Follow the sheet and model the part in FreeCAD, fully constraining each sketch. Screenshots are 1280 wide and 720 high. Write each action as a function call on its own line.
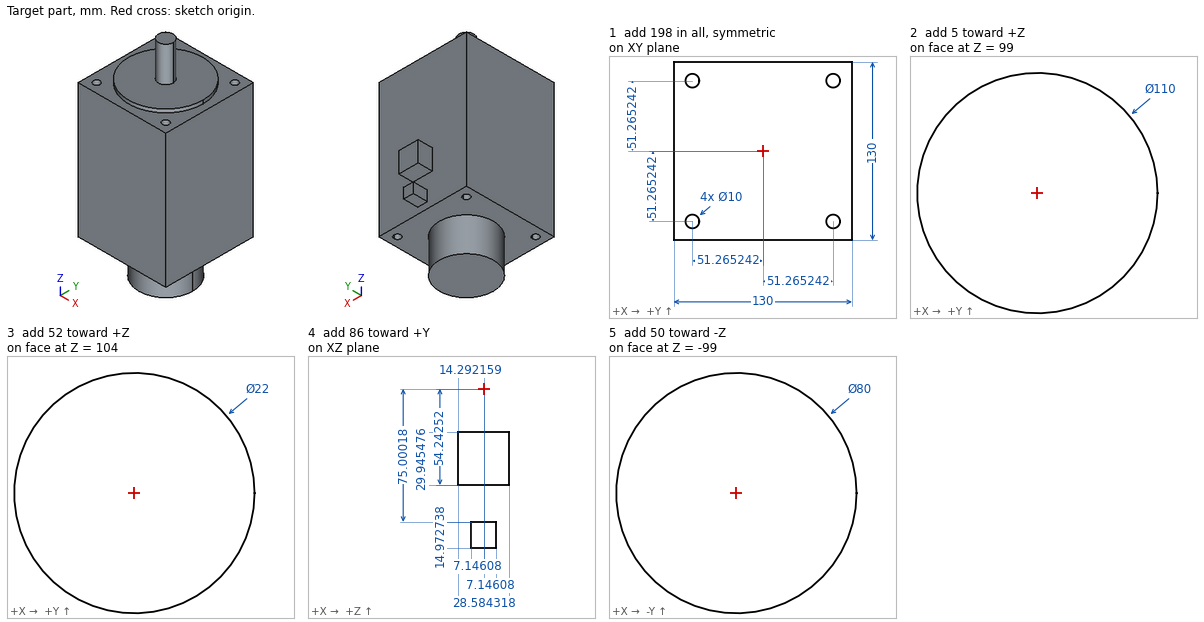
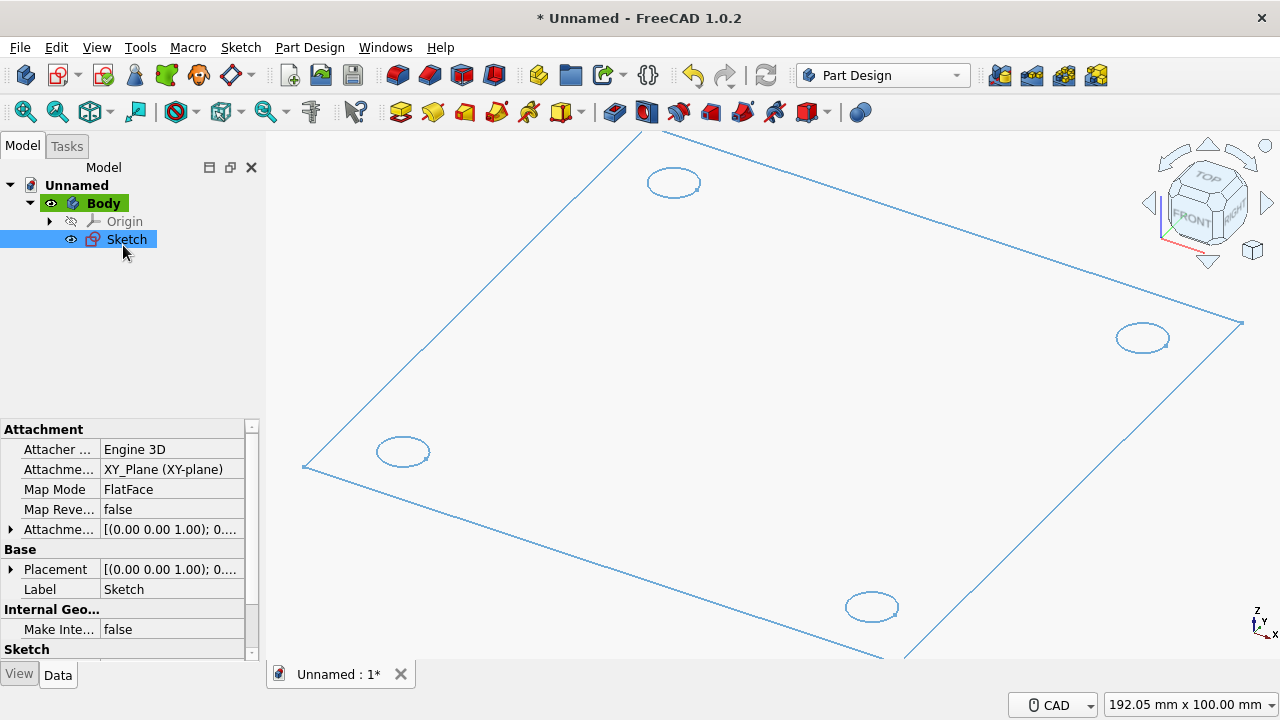
click(402, 112)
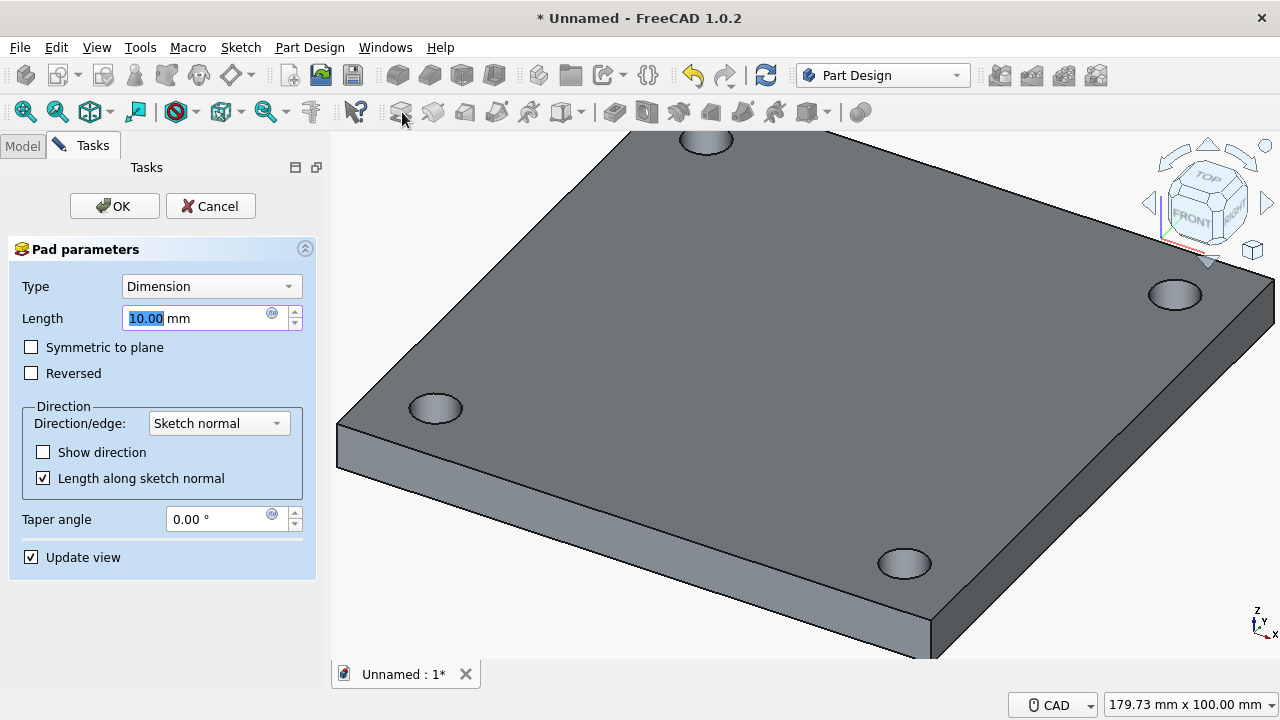
text(198)
key(Tab)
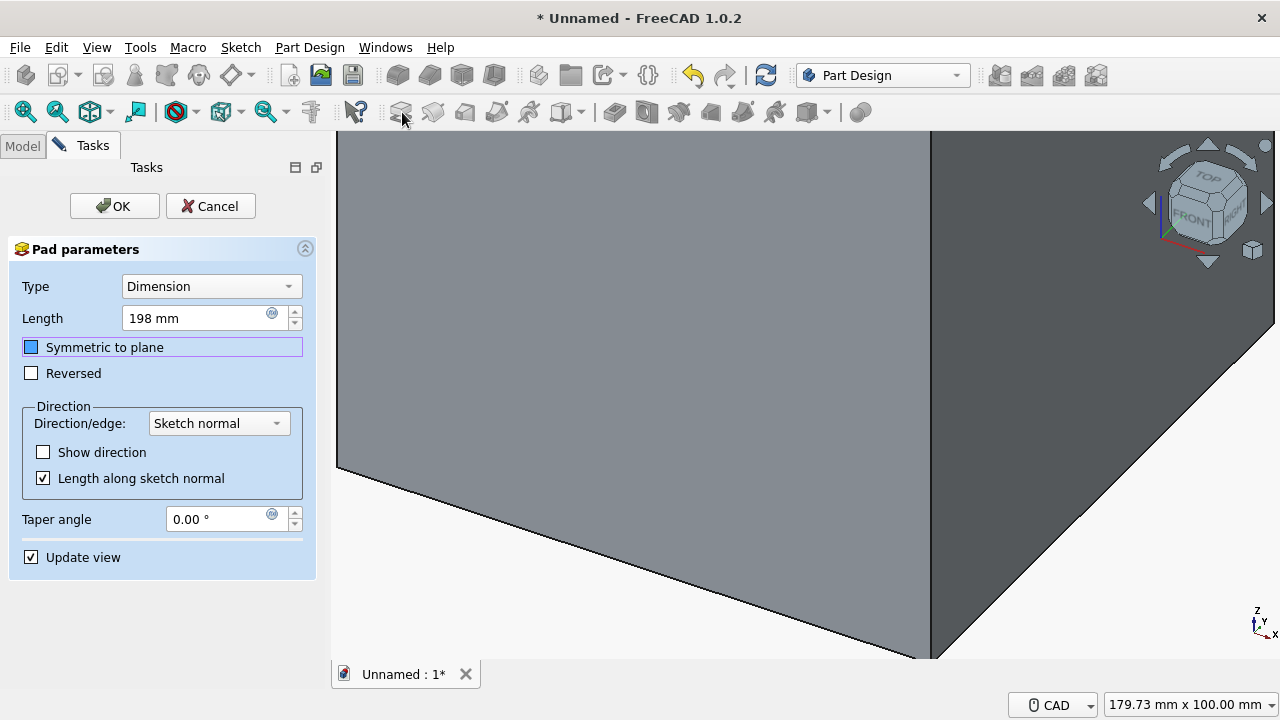
click(30, 347)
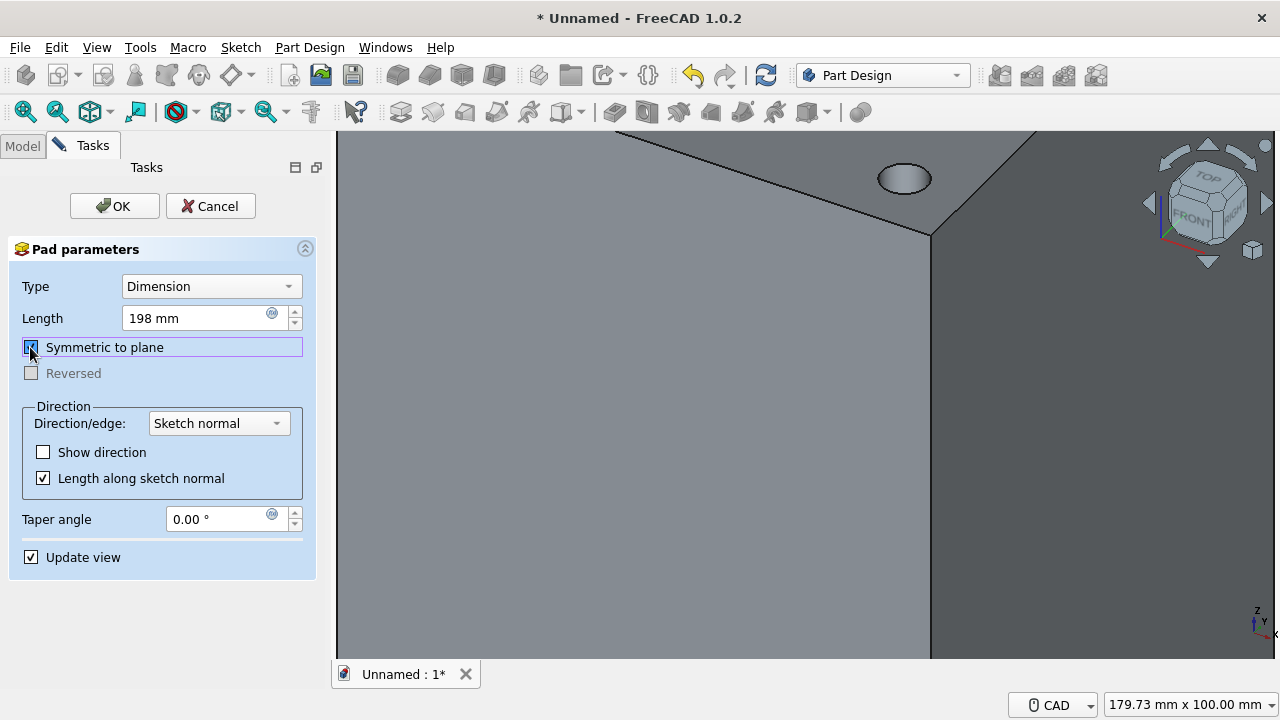
click(115, 206)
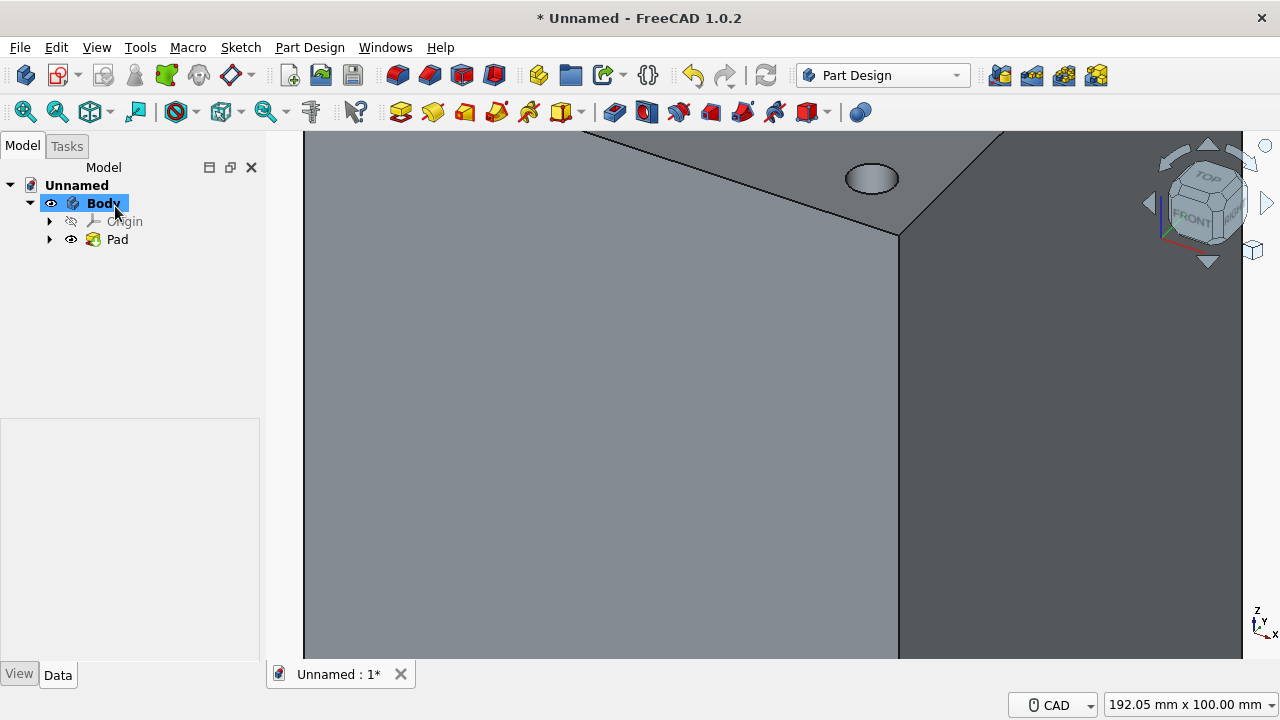
click(26, 112)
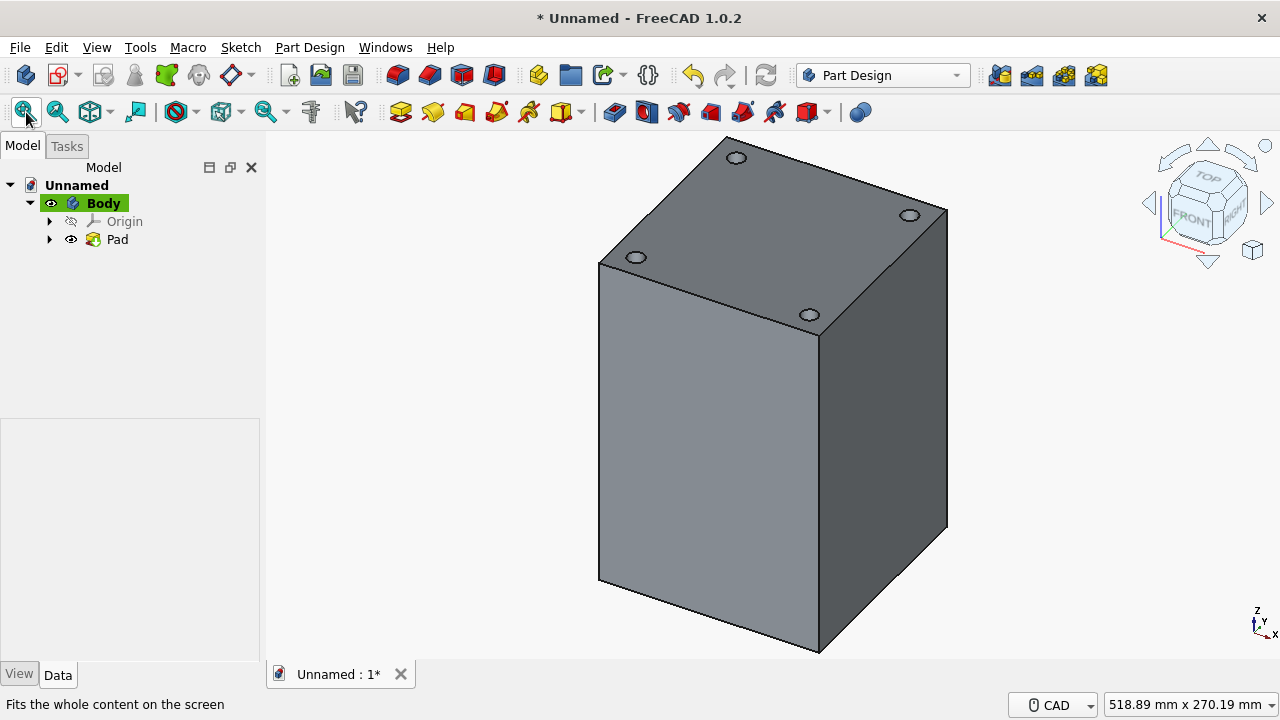
click(773, 236)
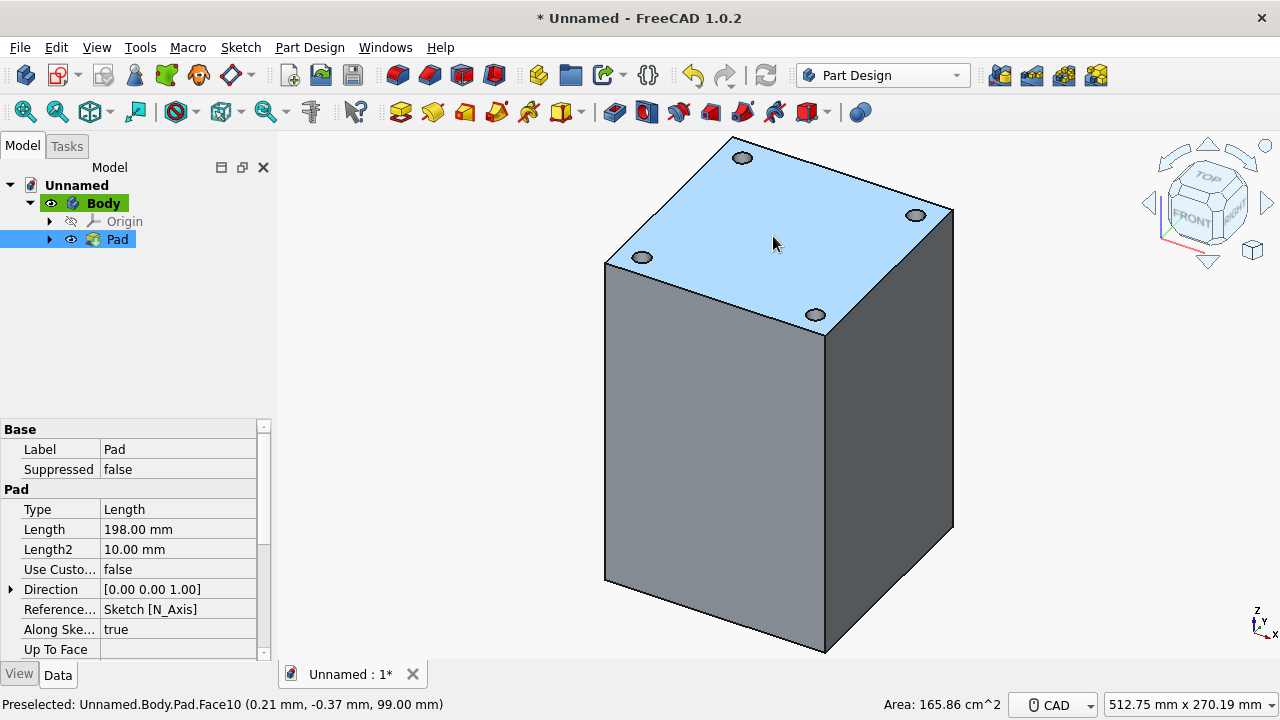
click(58, 76)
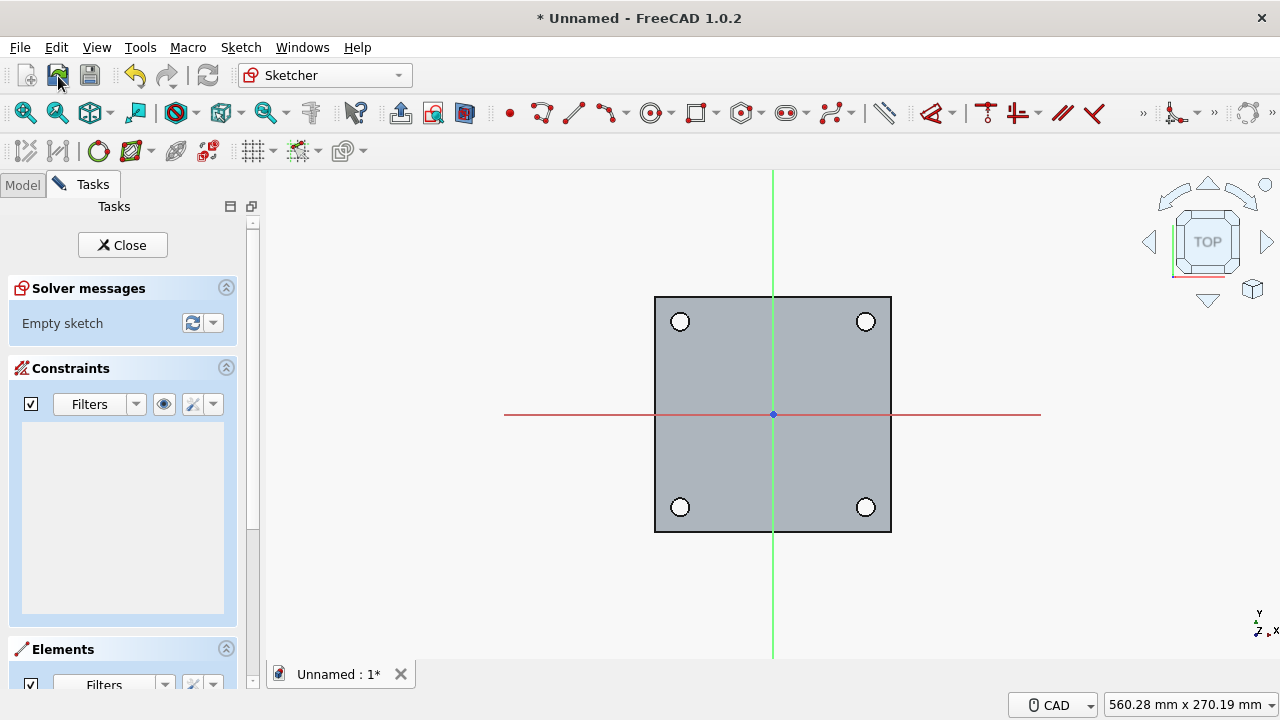
scroll(912, 414, up, 2)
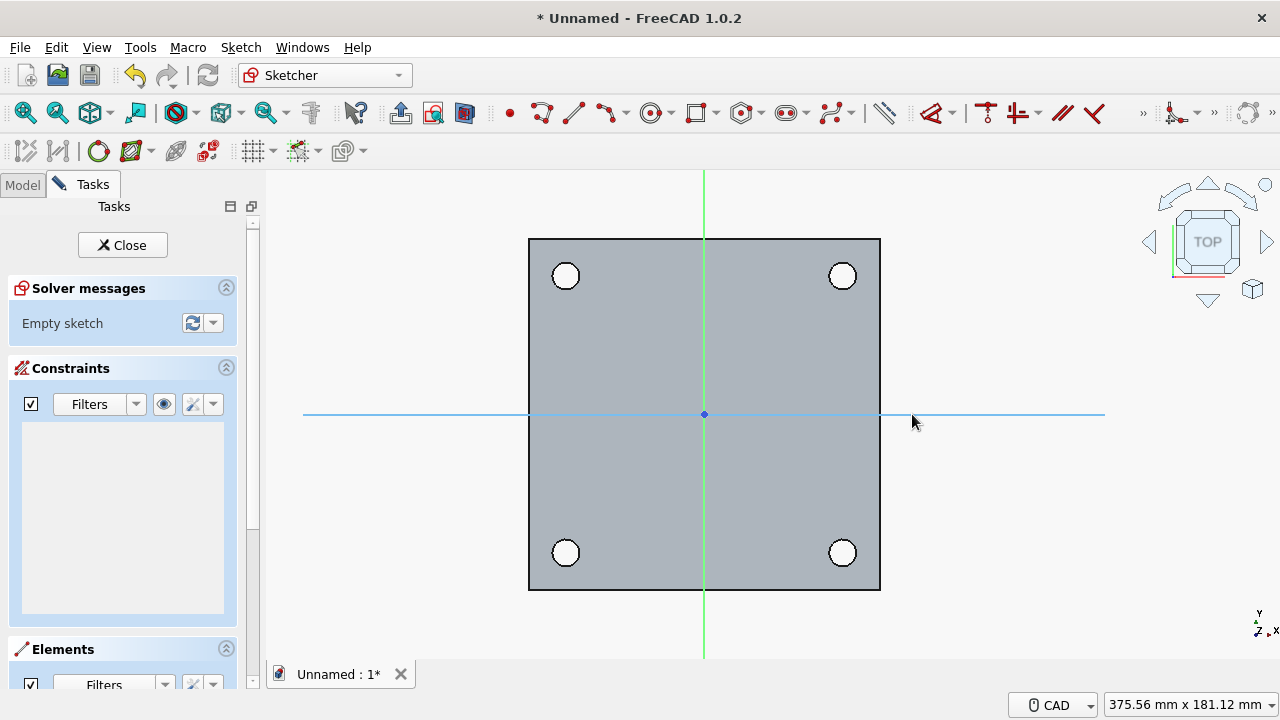
key(g)
key(c)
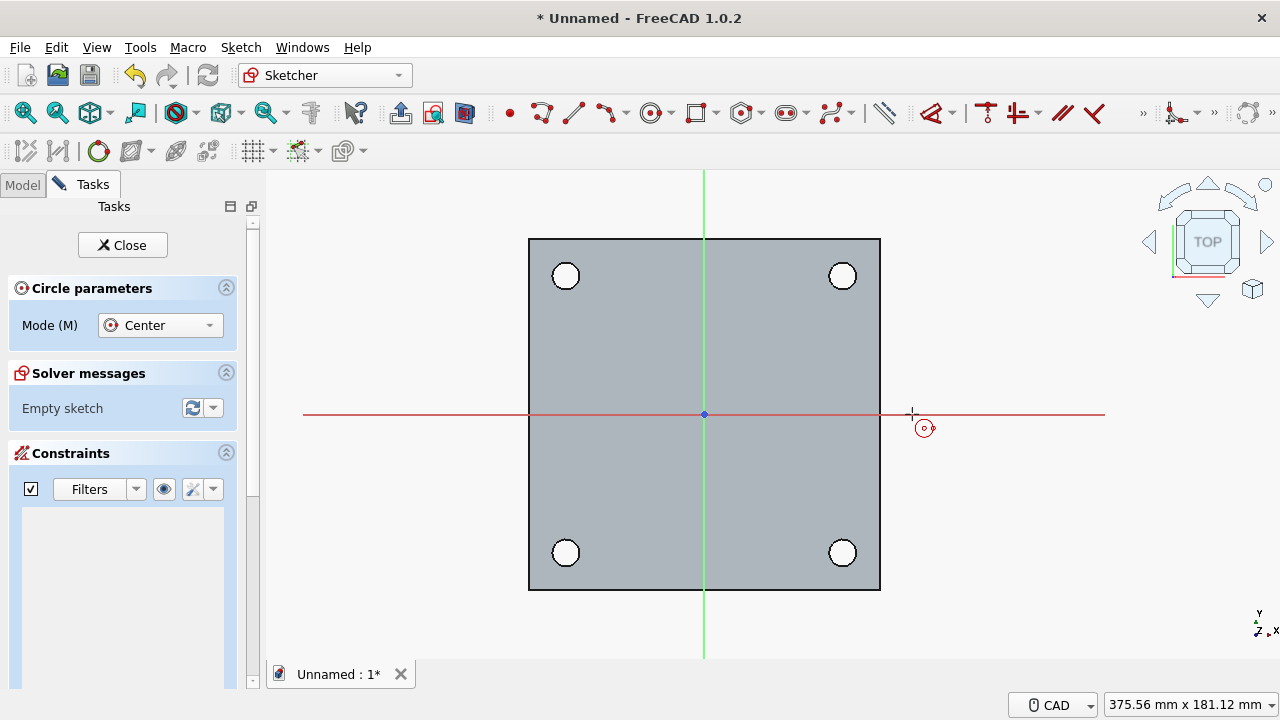
click(704, 414)
click(809, 309)
key(Escape)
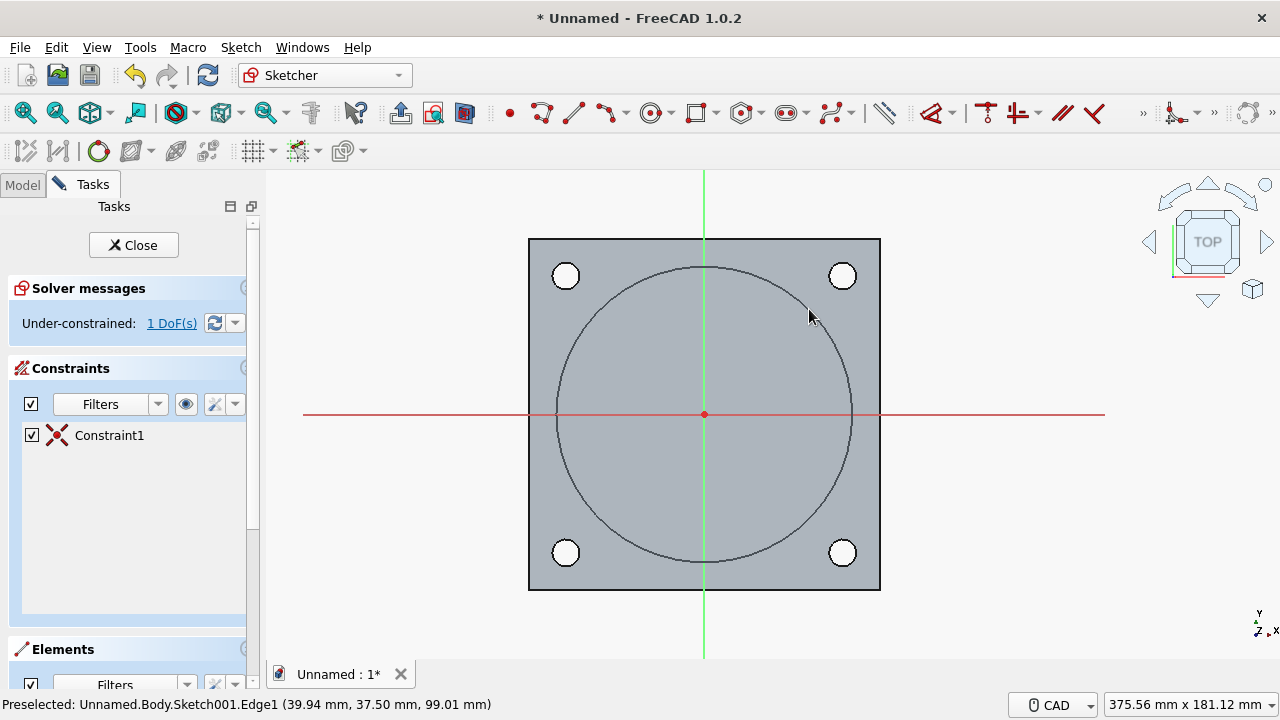
key(d)